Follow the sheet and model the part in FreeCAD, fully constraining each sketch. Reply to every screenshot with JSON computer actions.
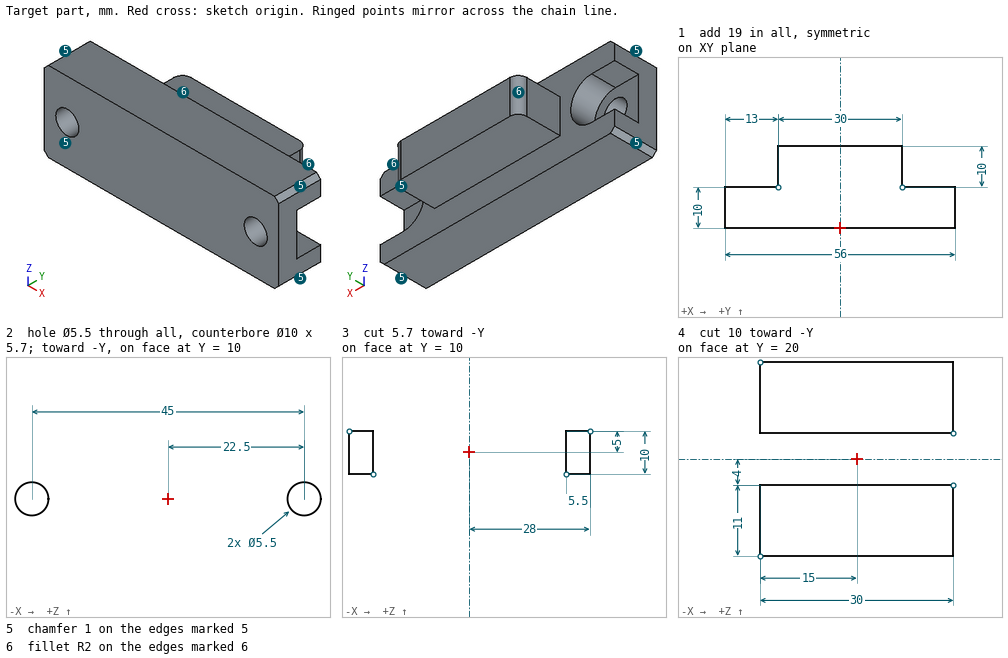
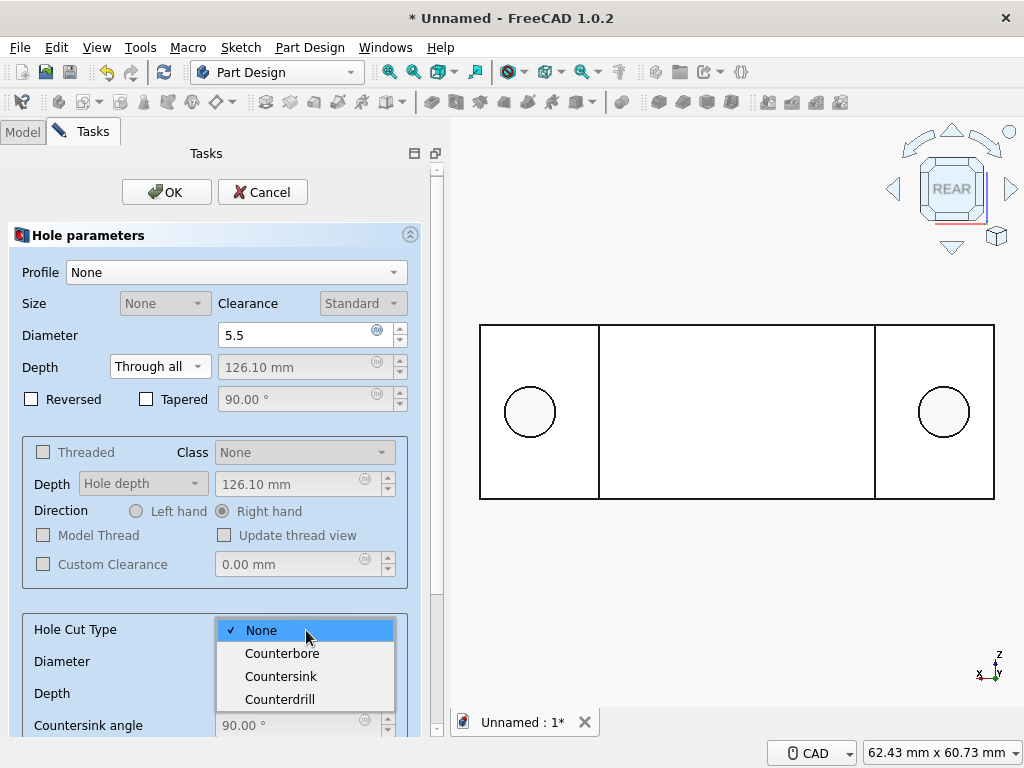
{"action": "left_click", "coordinate": [304, 654]}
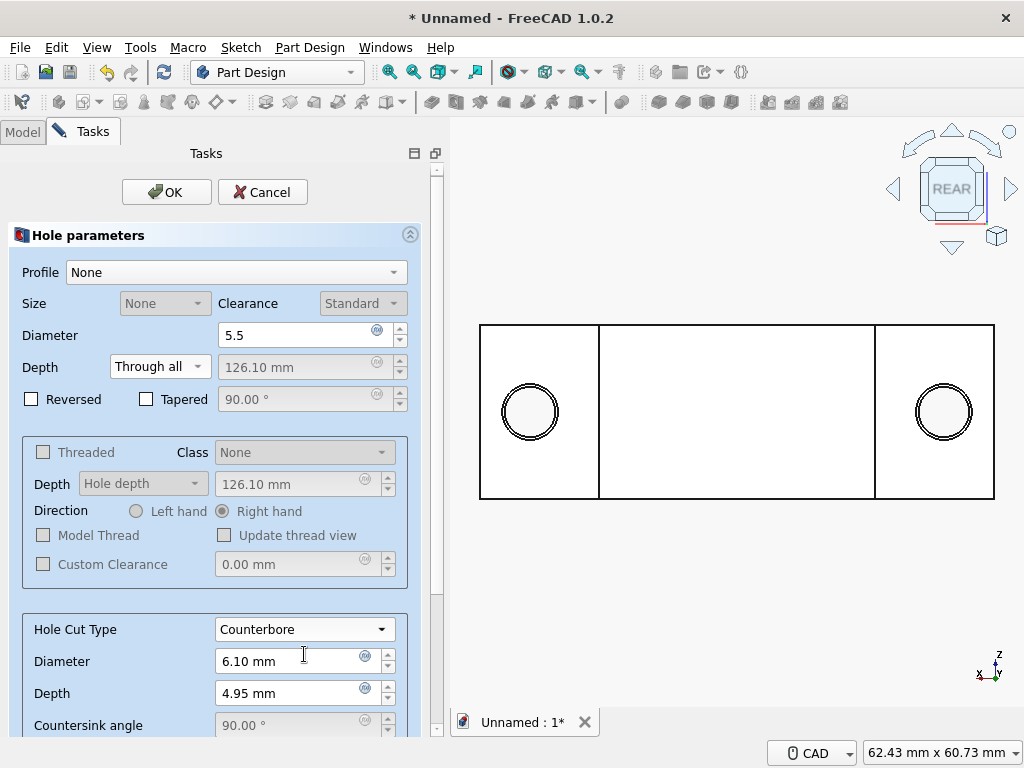
{"action": "triple_click", "coordinate": [298, 661]}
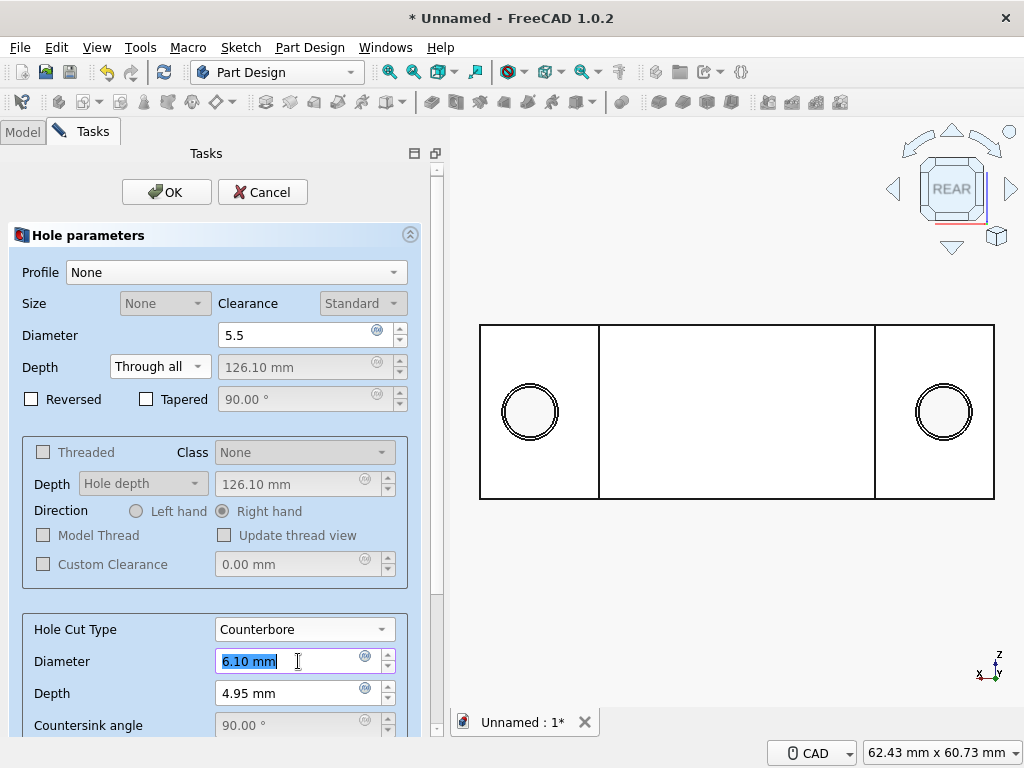
{"action": "type", "text": "10"}
{"action": "key", "text": "Tab"}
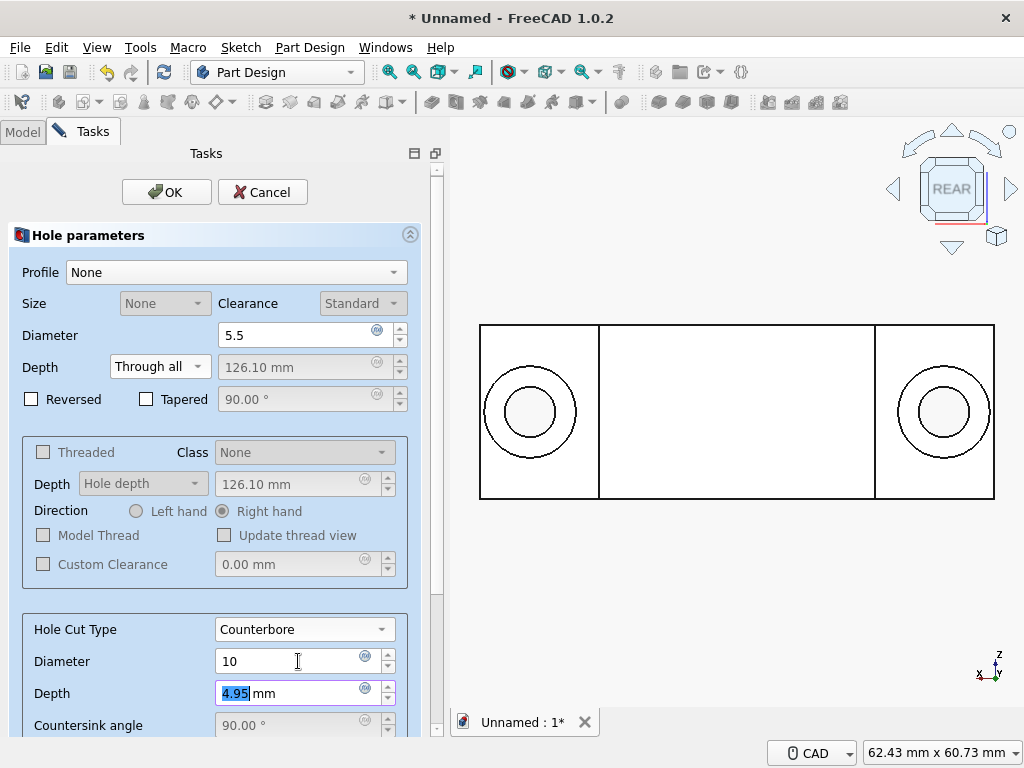
{"action": "type", "text": "5.7"}
{"action": "key", "text": "Tab"}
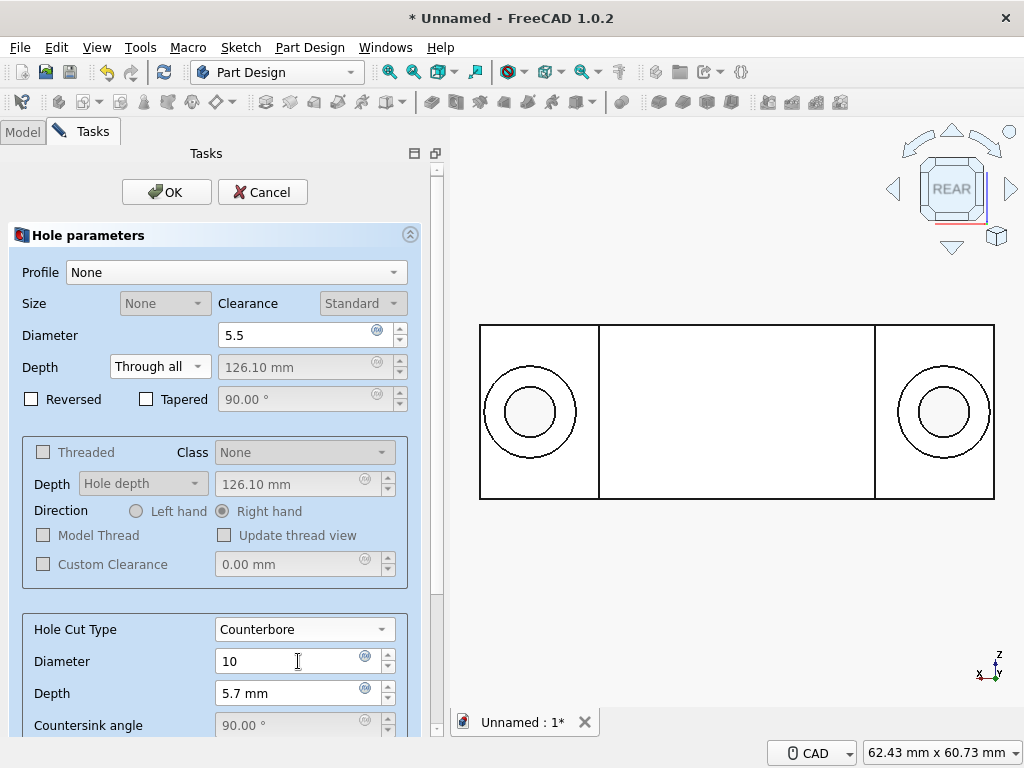
{"action": "left_click", "coordinate": [167, 192]}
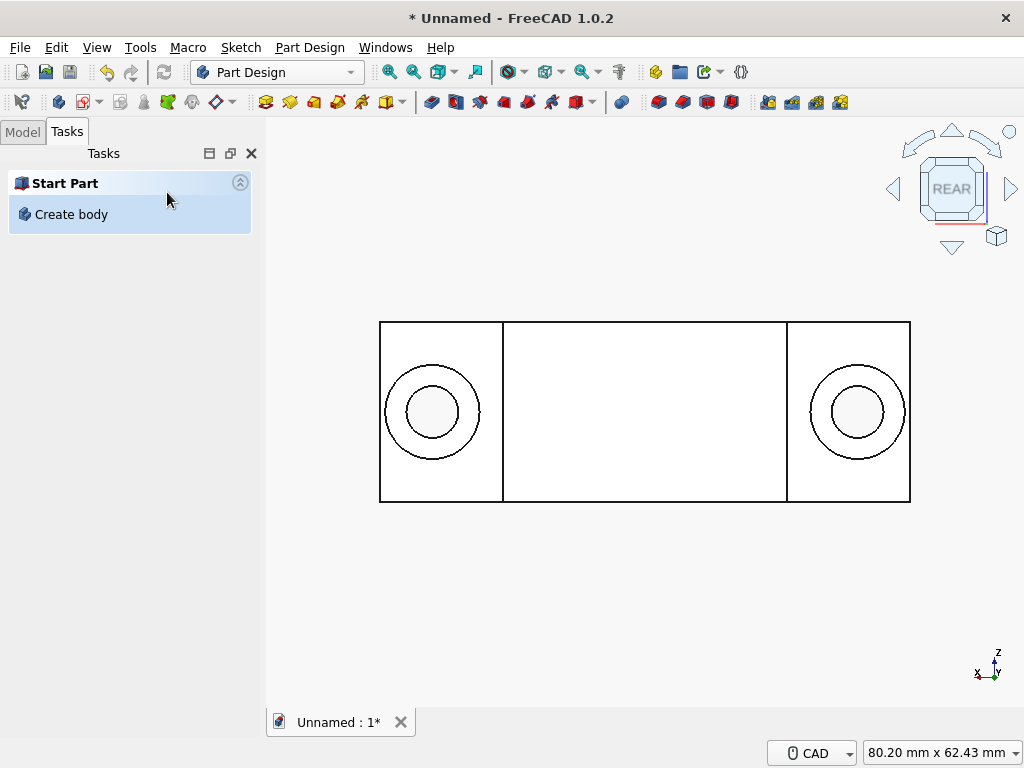
{"action": "left_click", "coordinate": [813, 360]}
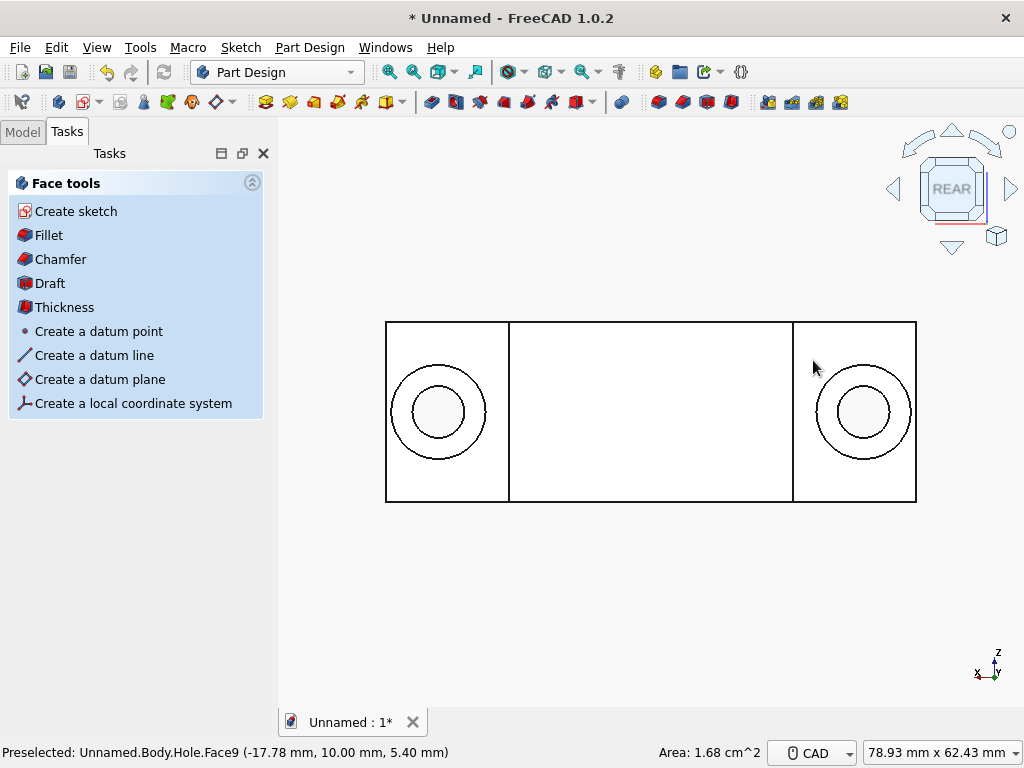
{"action": "left_click", "coordinate": [84, 102]}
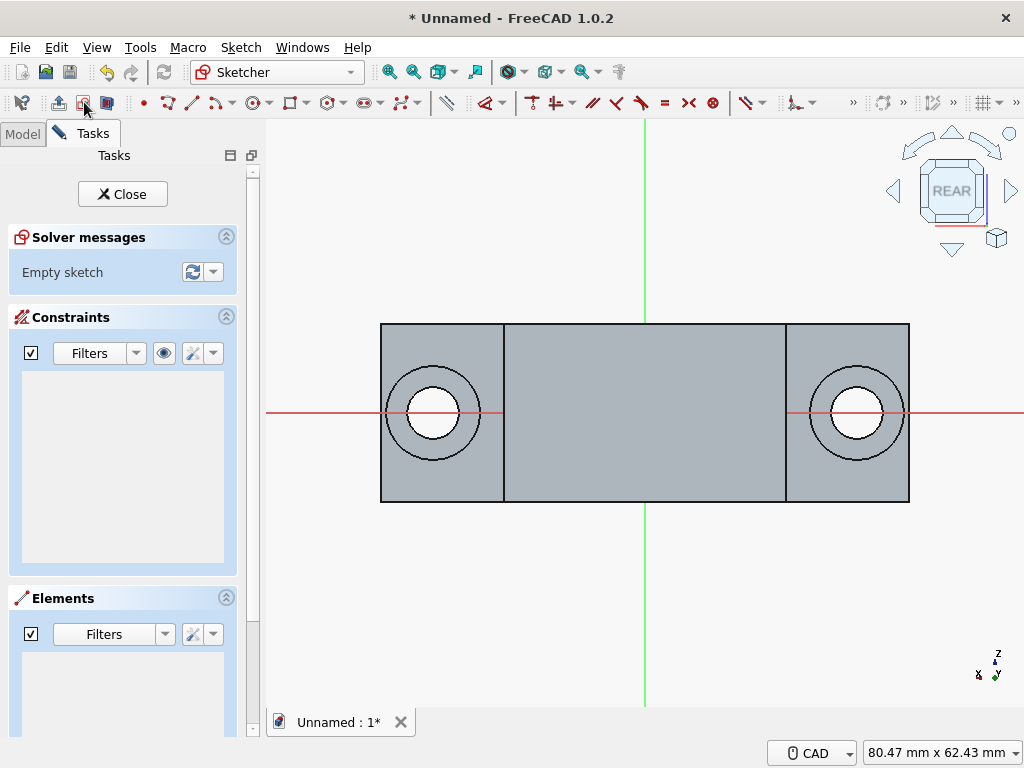
{"action": "key", "text": "q s"}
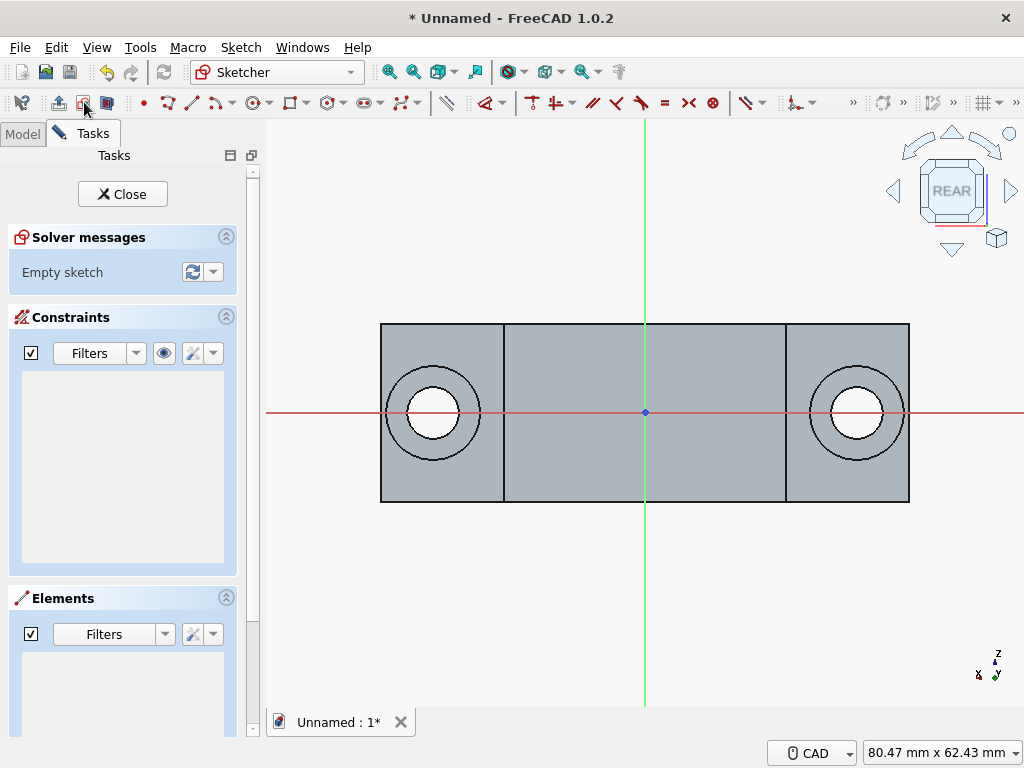
{"action": "scroll", "coordinate": [294, 413], "scroll_direction": "down", "scroll_amount": 1}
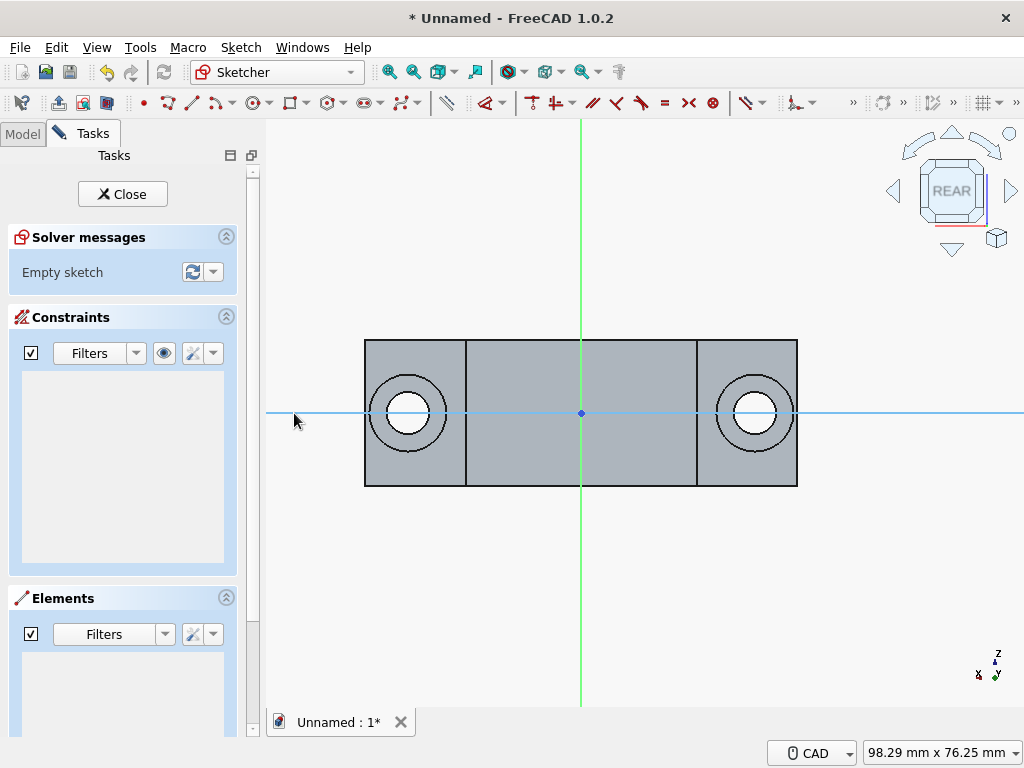
{"action": "key", "text": "g r"}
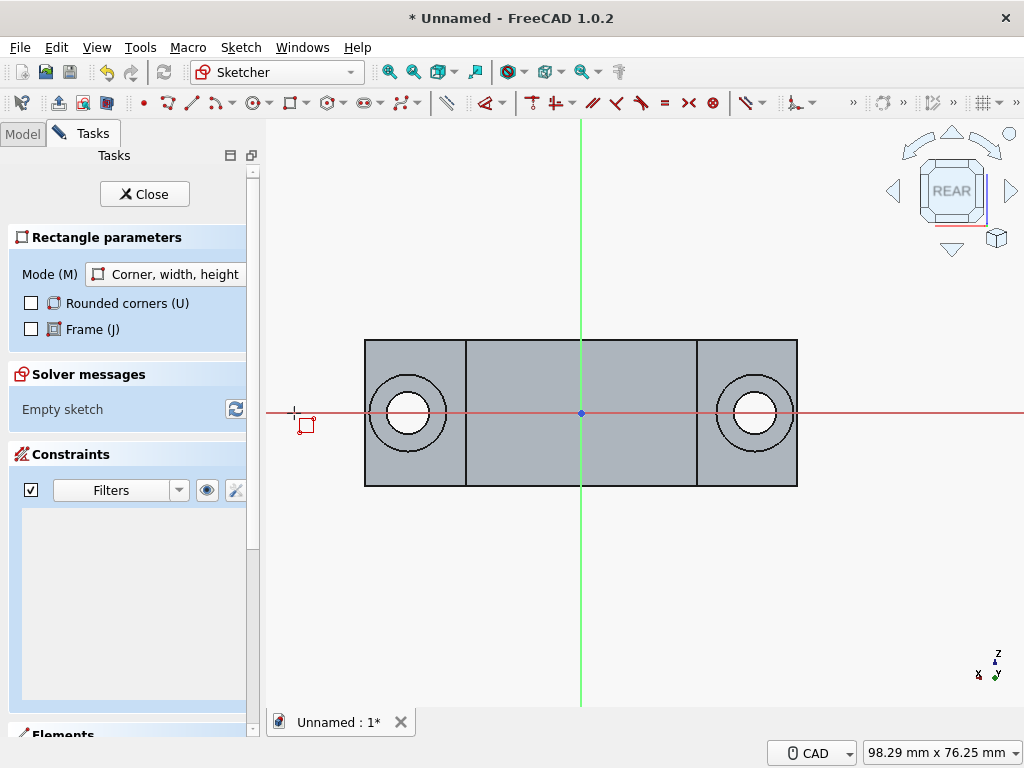
{"action": "left_click", "coordinate": [755, 375]}
{"action": "left_click", "coordinate": [797, 452]}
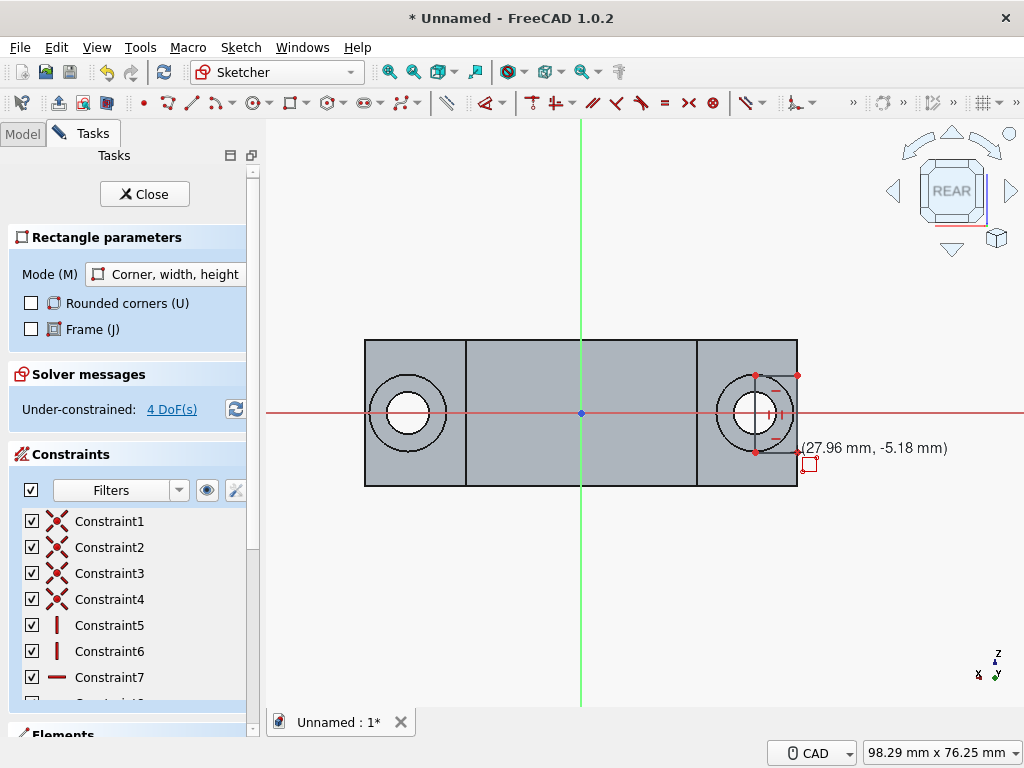
{"action": "left_click", "coordinate": [365, 375]}
{"action": "left_click", "coordinate": [408, 452]}
{"action": "key", "text": "Escape"}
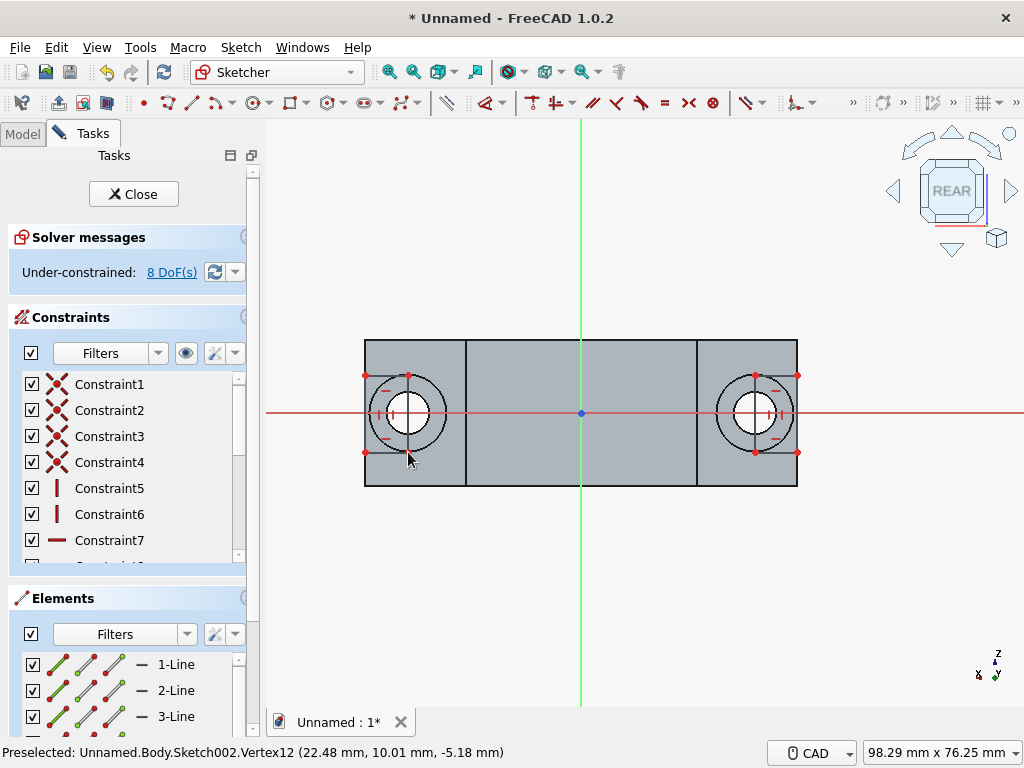
{"action": "left_click", "coordinate": [797, 376]}